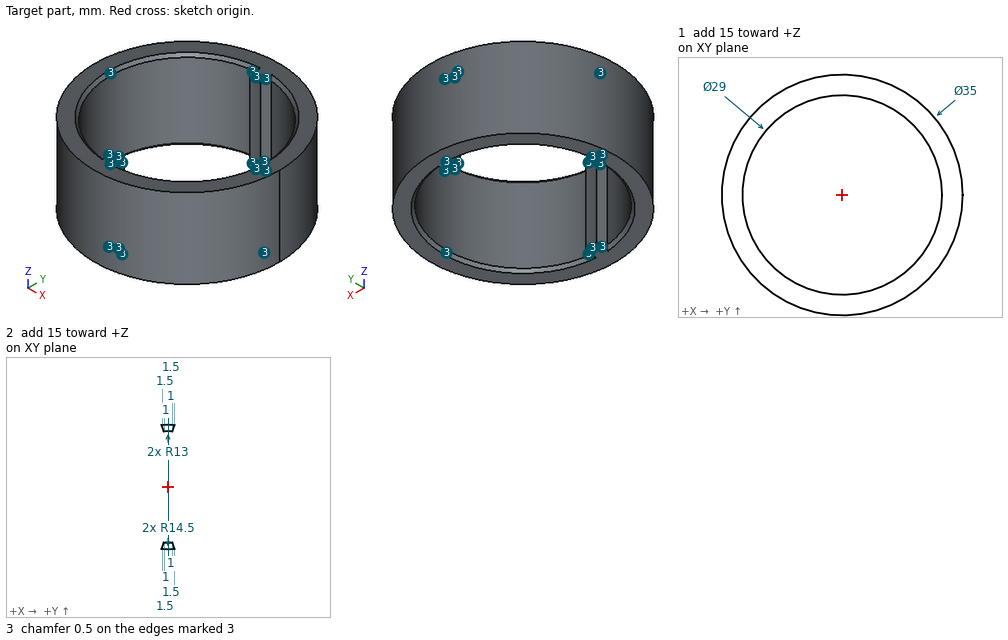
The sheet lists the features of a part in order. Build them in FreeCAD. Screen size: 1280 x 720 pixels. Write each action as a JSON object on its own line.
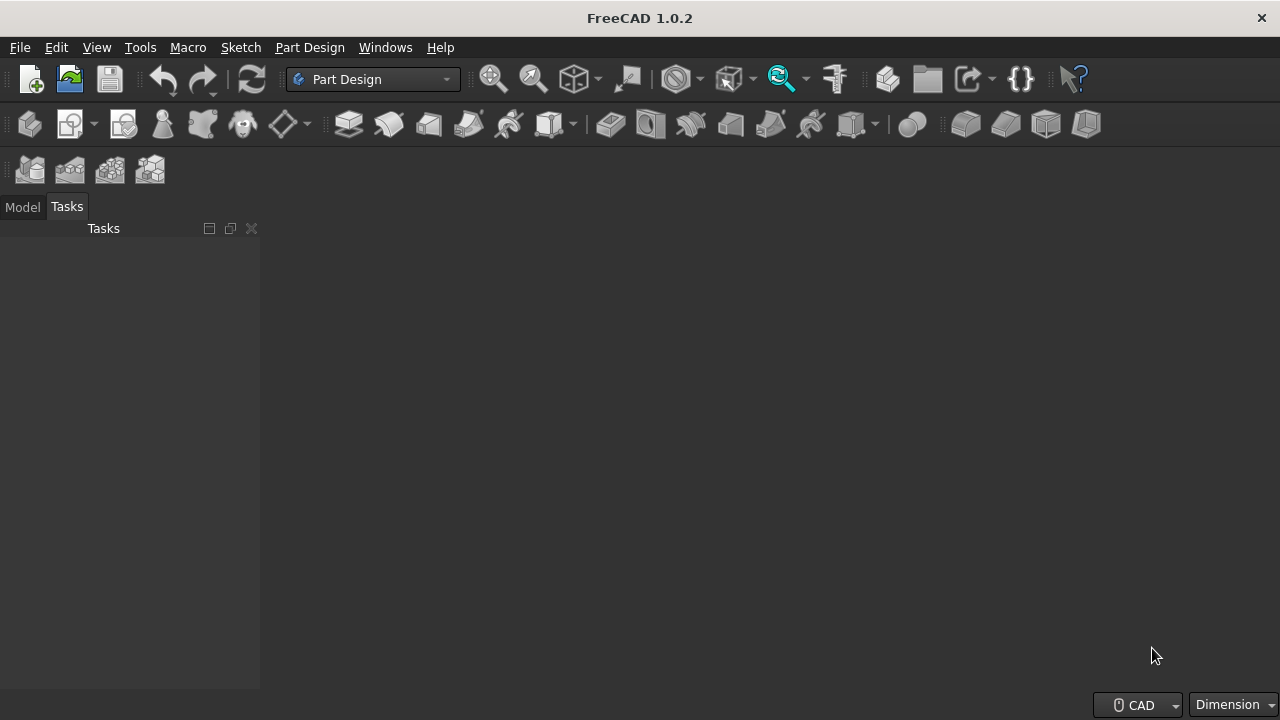
{"action": "left_click", "coordinate": [30, 80]}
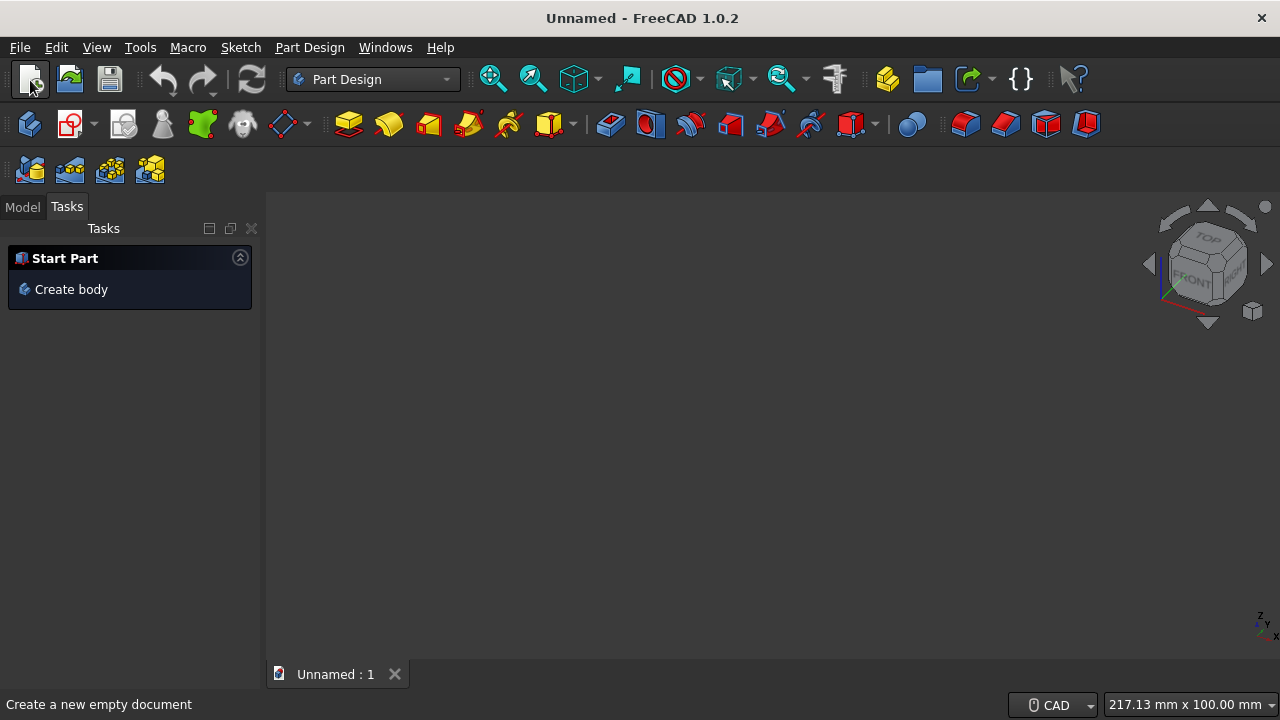
{"action": "left_click", "coordinate": [70, 124]}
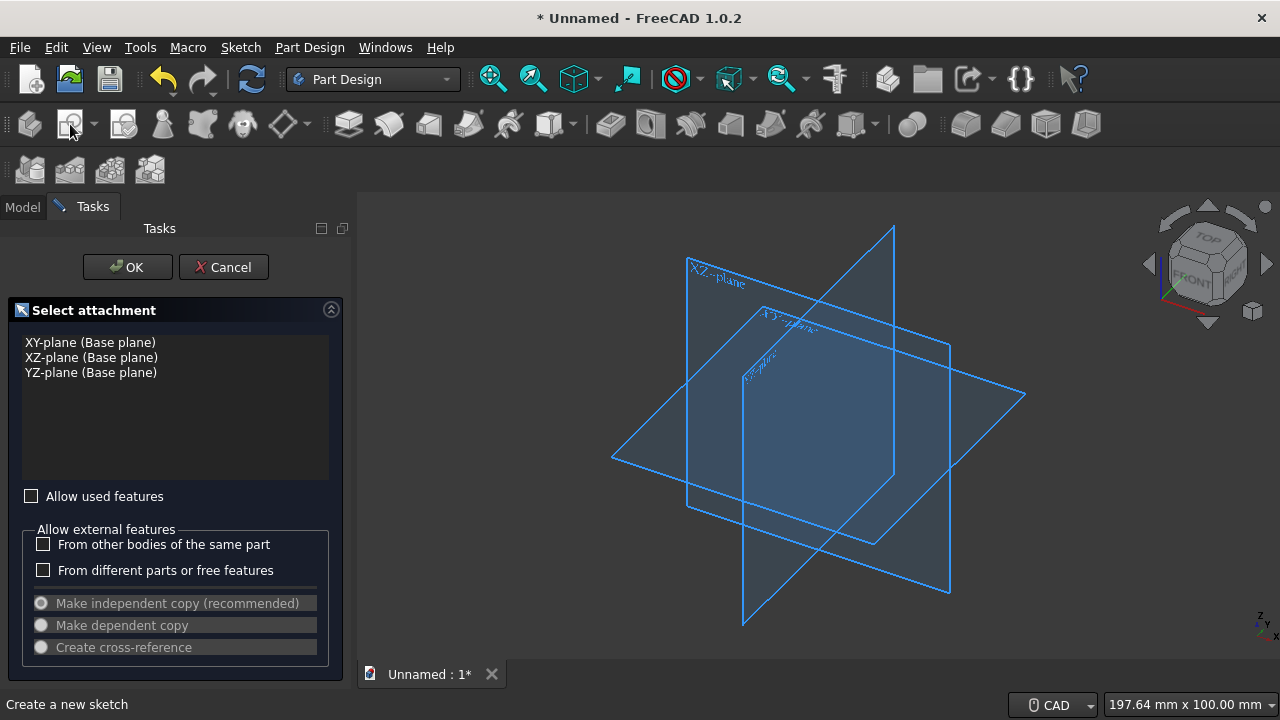
{"action": "left_click", "coordinate": [82, 342]}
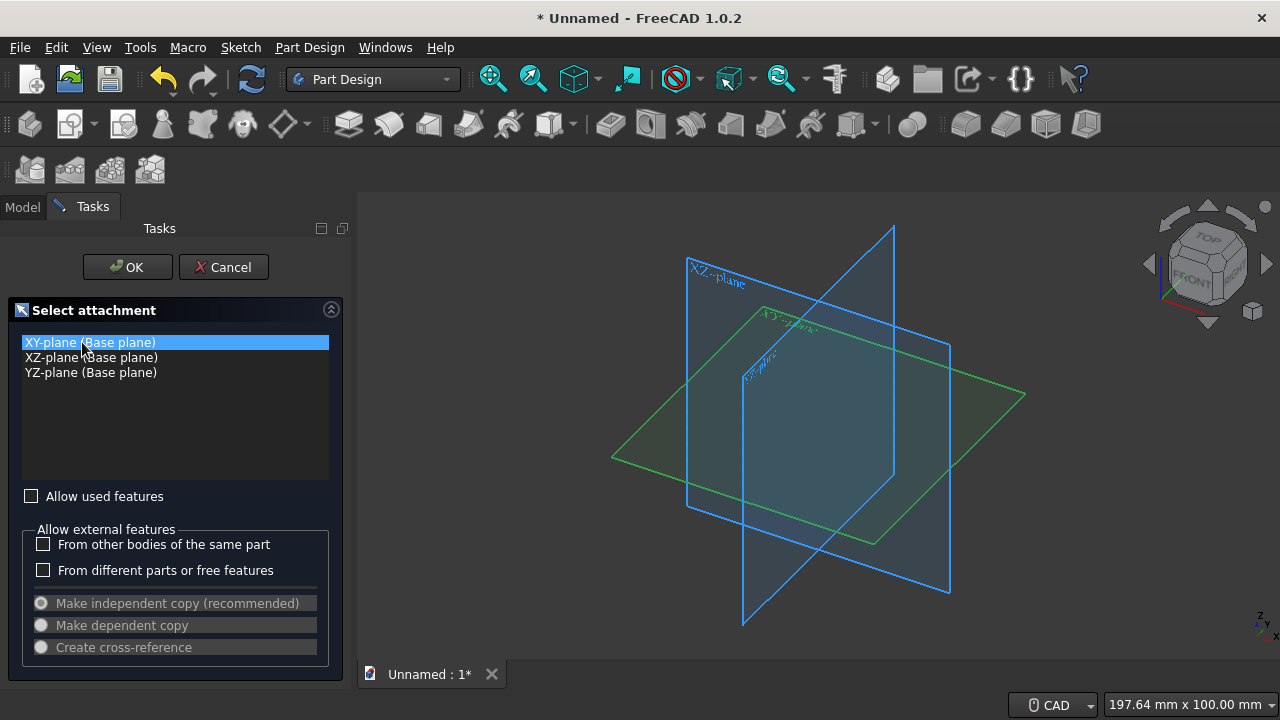
{"action": "left_click", "coordinate": [128, 267]}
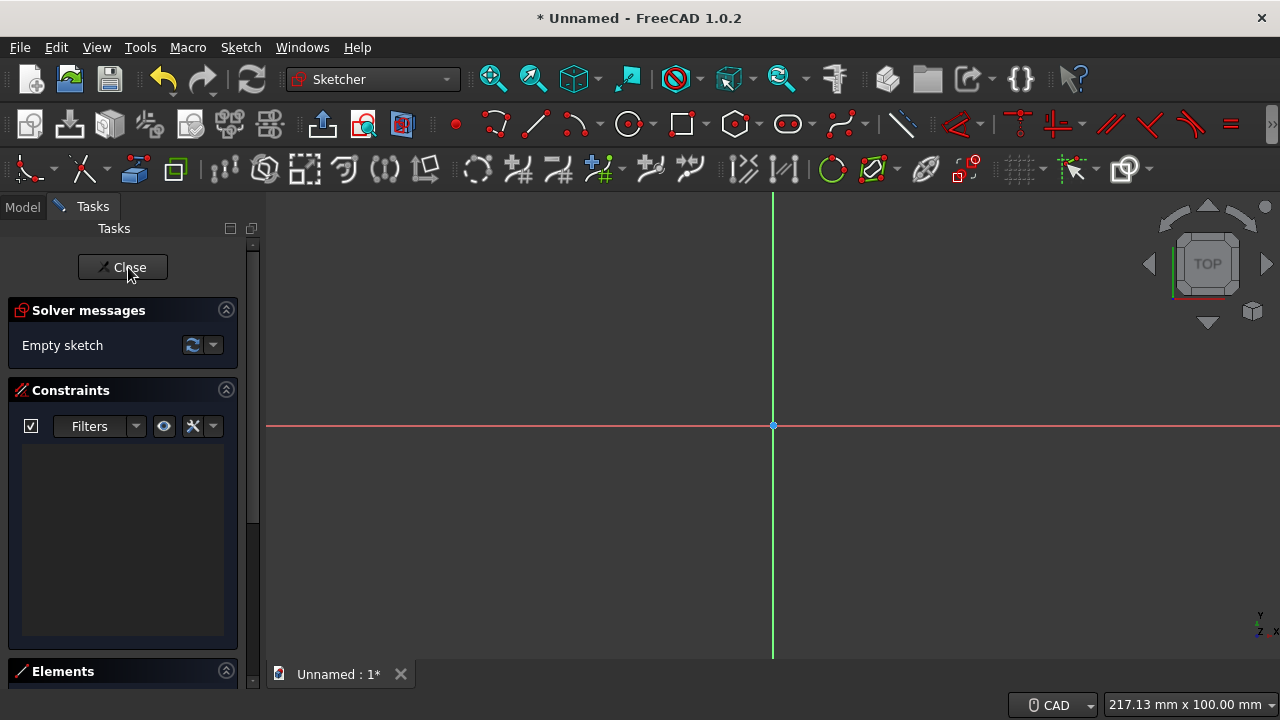
{"action": "scroll", "coordinate": [856, 426], "scroll_direction": "up", "scroll_amount": 3}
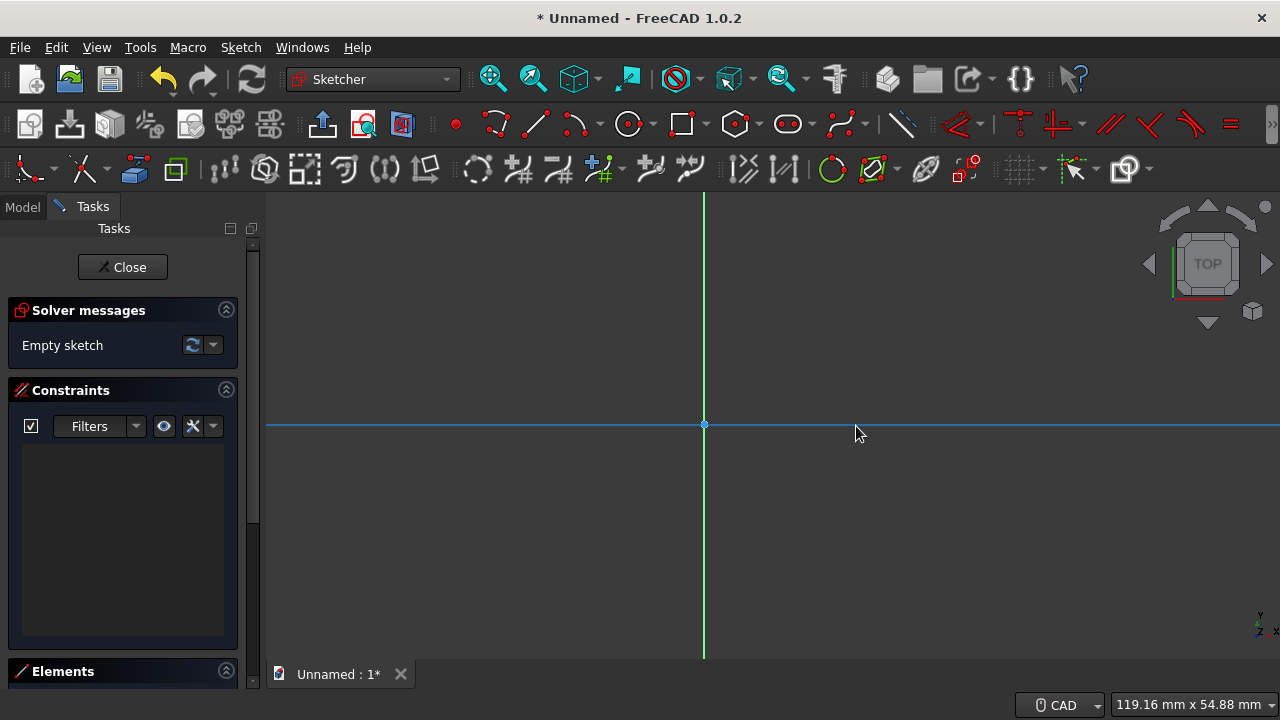
{"action": "key", "text": "g c"}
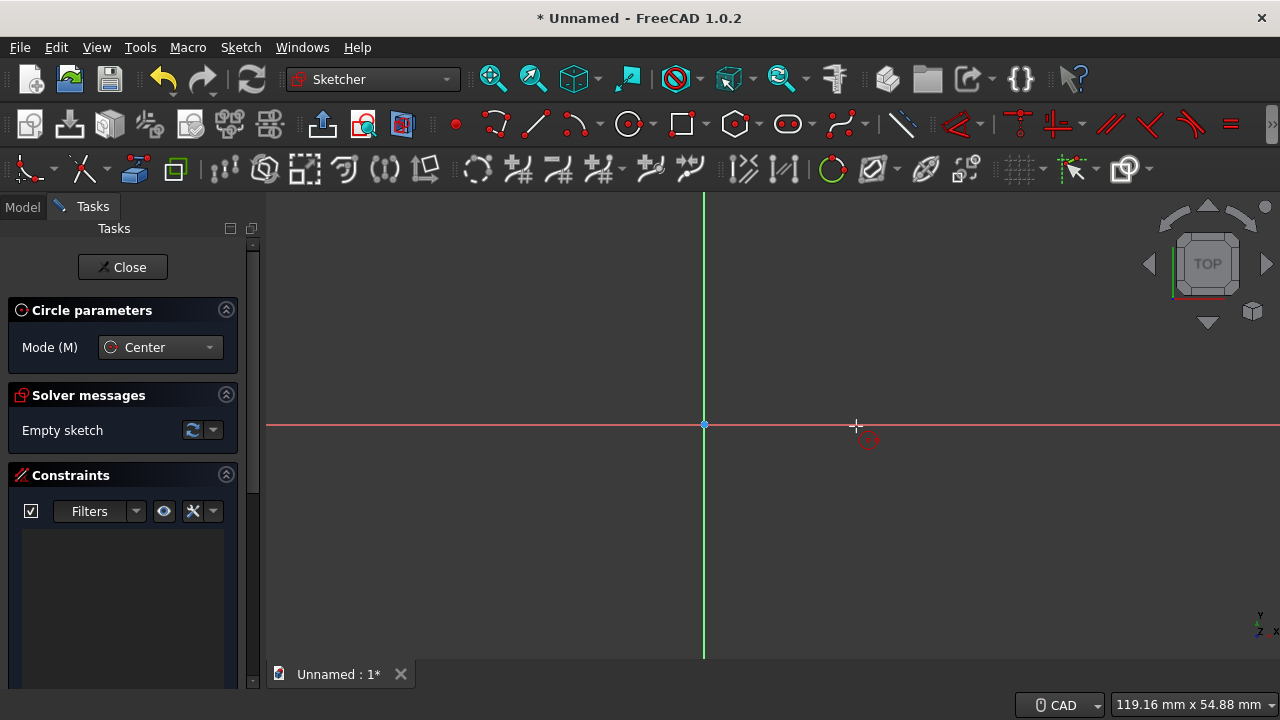
{"action": "left_click", "coordinate": [704, 425]}
{"action": "left_click", "coordinate": [810, 319]}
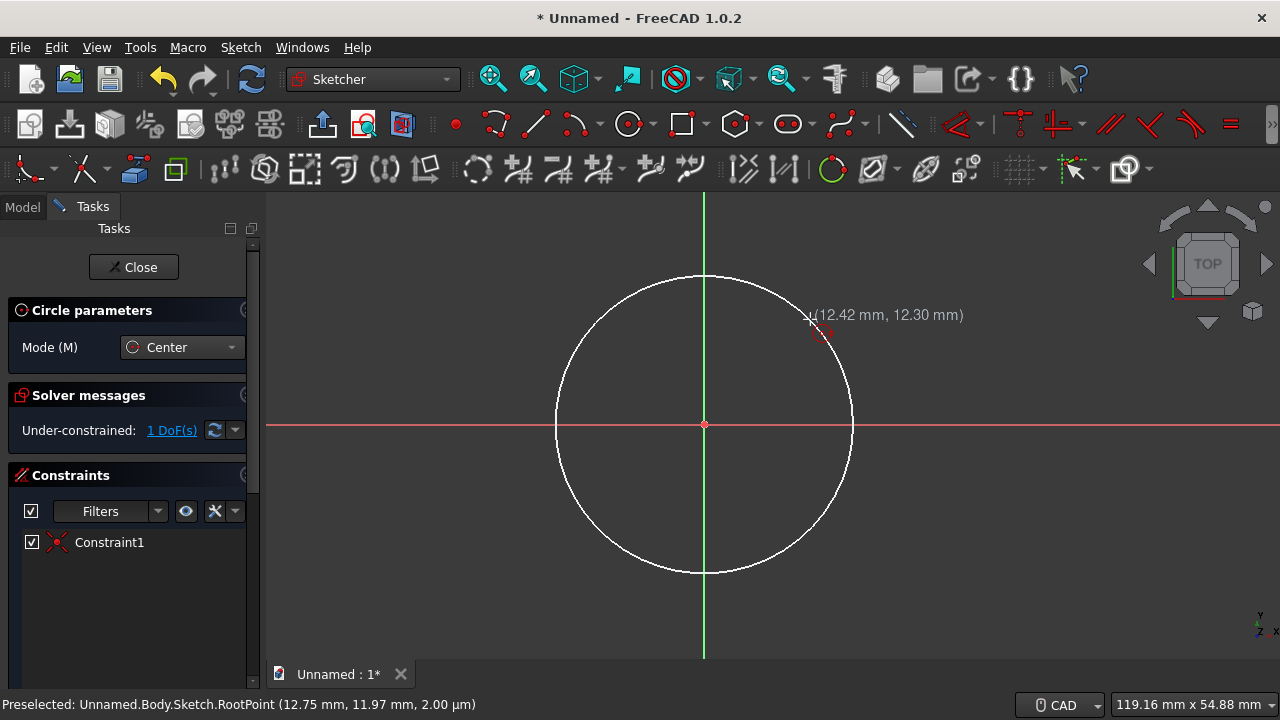
{"action": "left_click", "coordinate": [704, 425]}
{"action": "left_click", "coordinate": [792, 337]}
{"action": "key", "text": "Escape"}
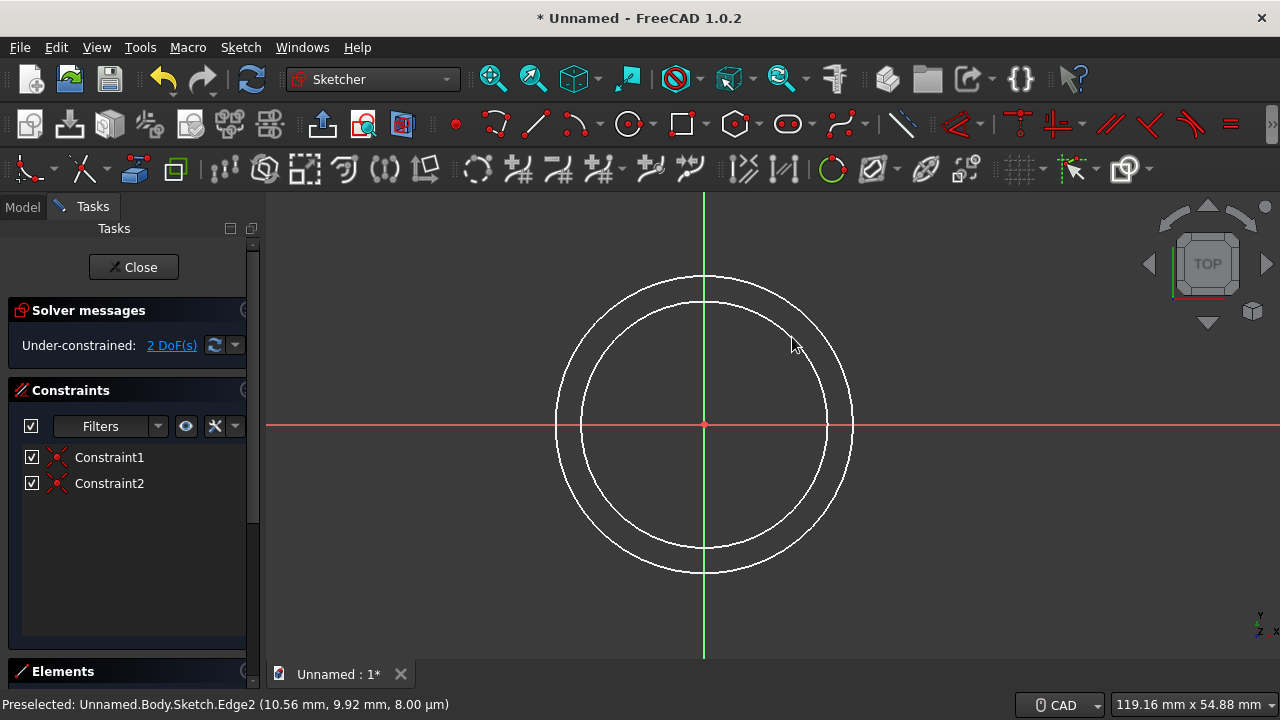
{"action": "left_click", "coordinate": [956, 124]}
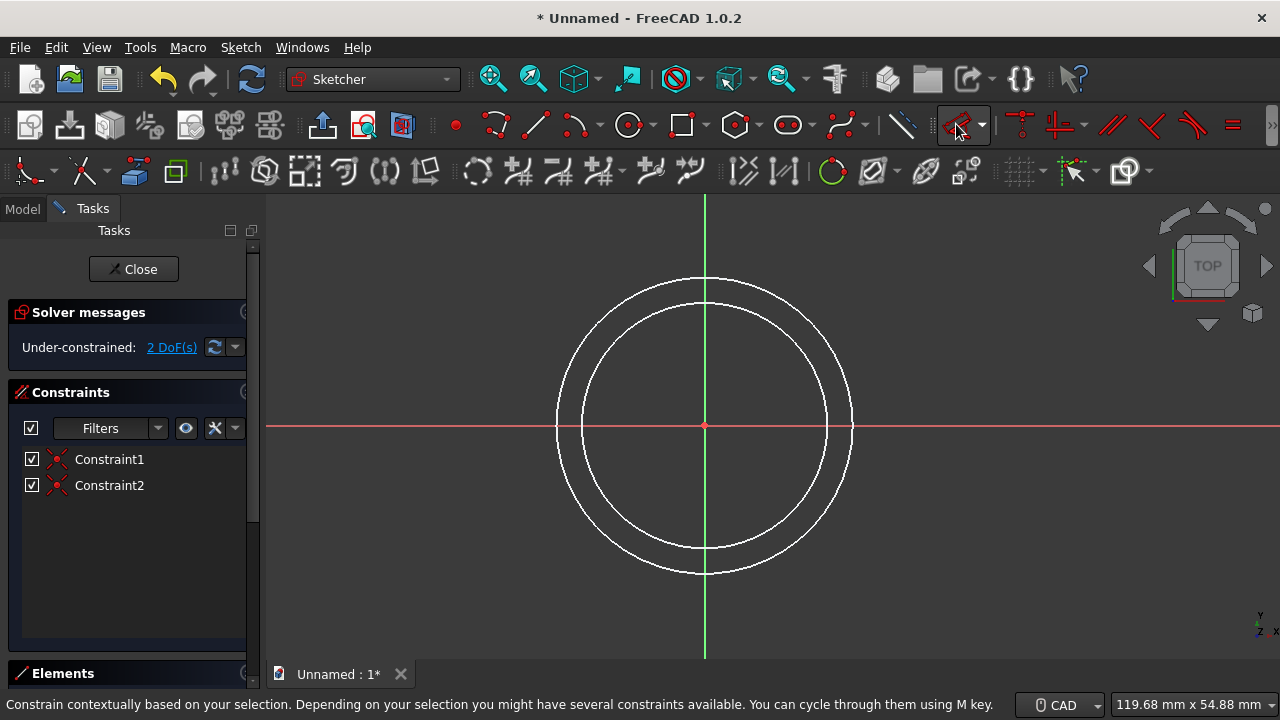
{"action": "left_click", "coordinate": [809, 321]}
{"action": "left_click", "coordinate": [832, 298]}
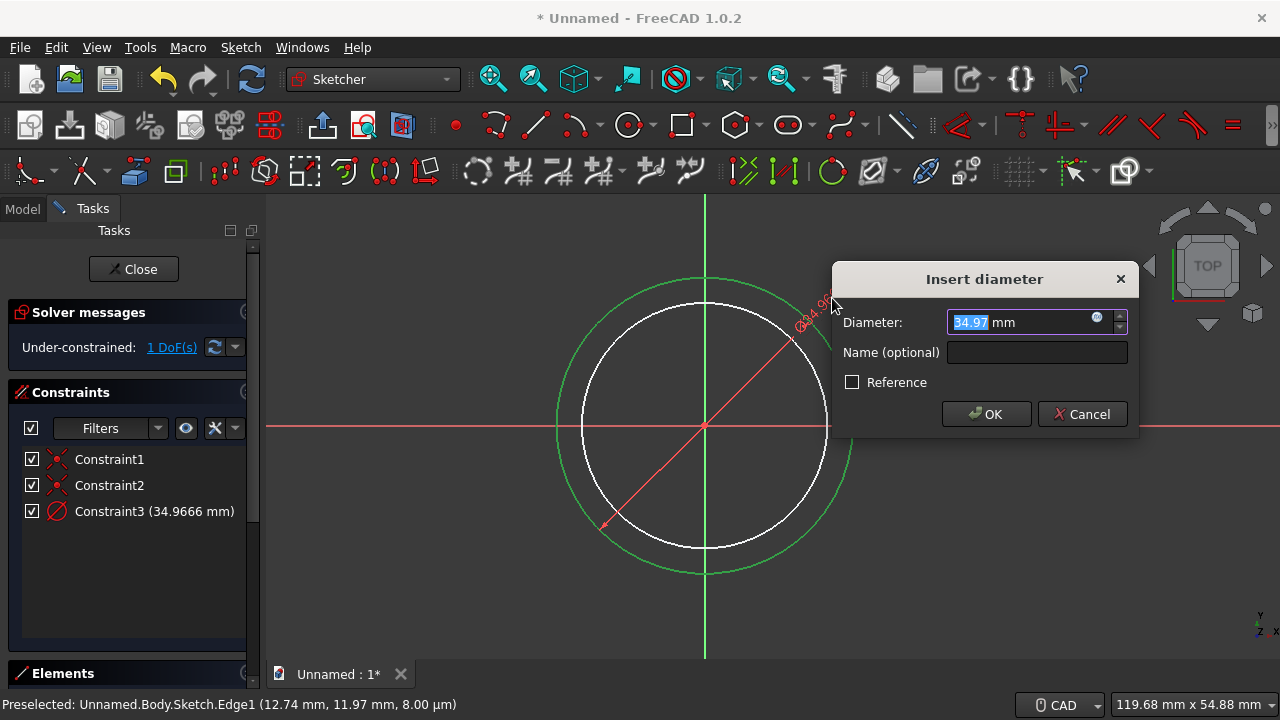
{"action": "type", "text": "35"}
{"action": "key", "text": "Return"}